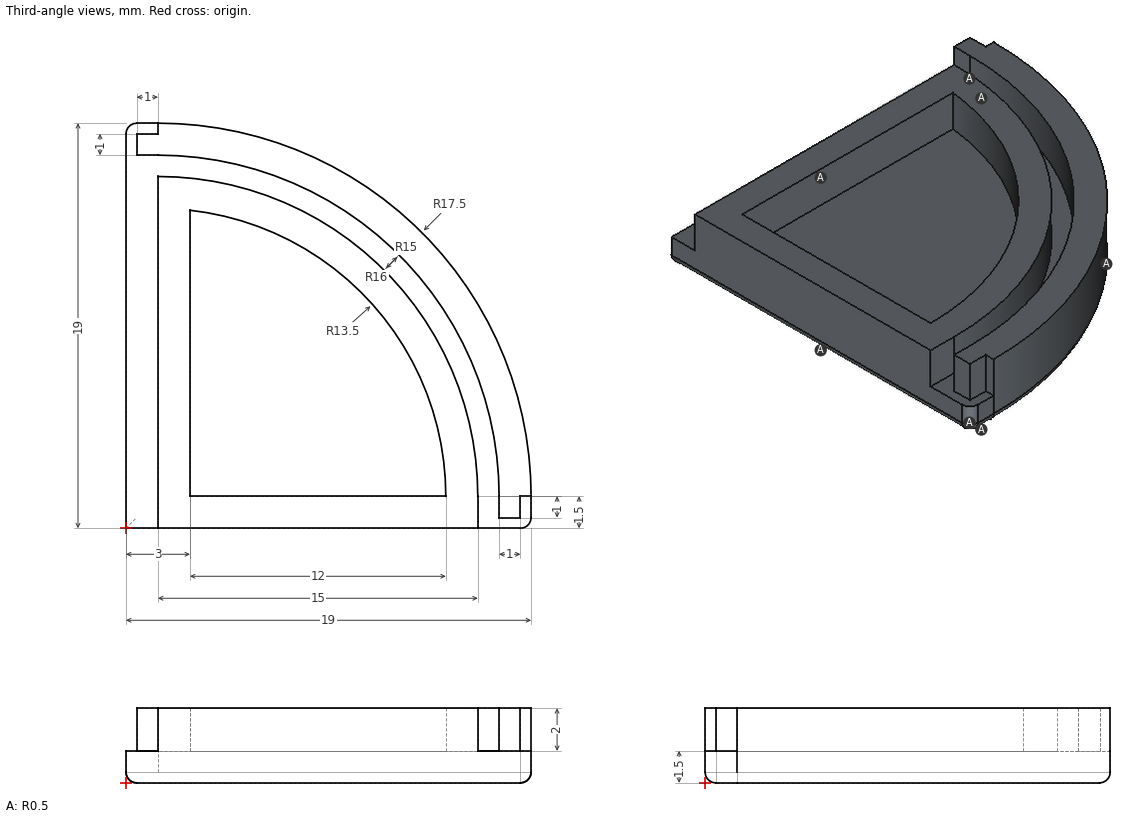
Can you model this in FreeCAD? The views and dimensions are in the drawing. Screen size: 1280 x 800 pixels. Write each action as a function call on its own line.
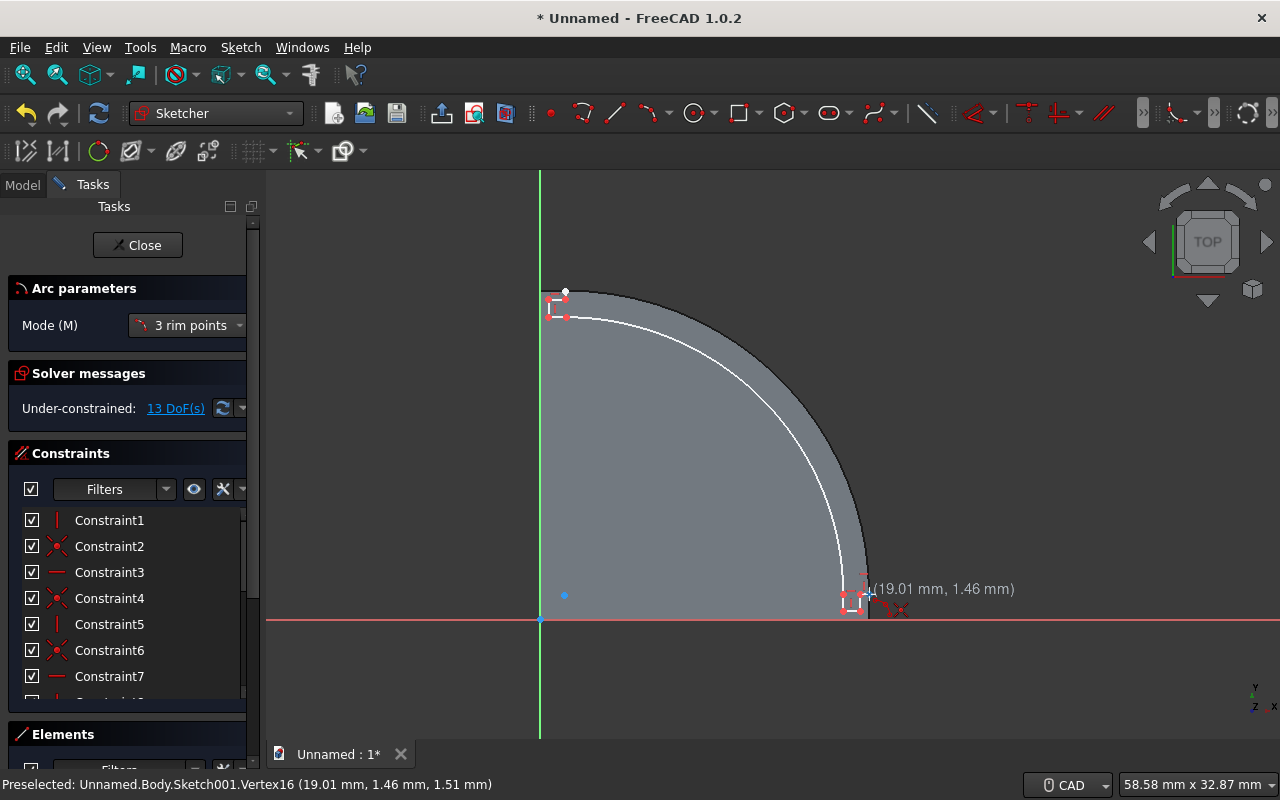
scroll(566, 291, up, 7)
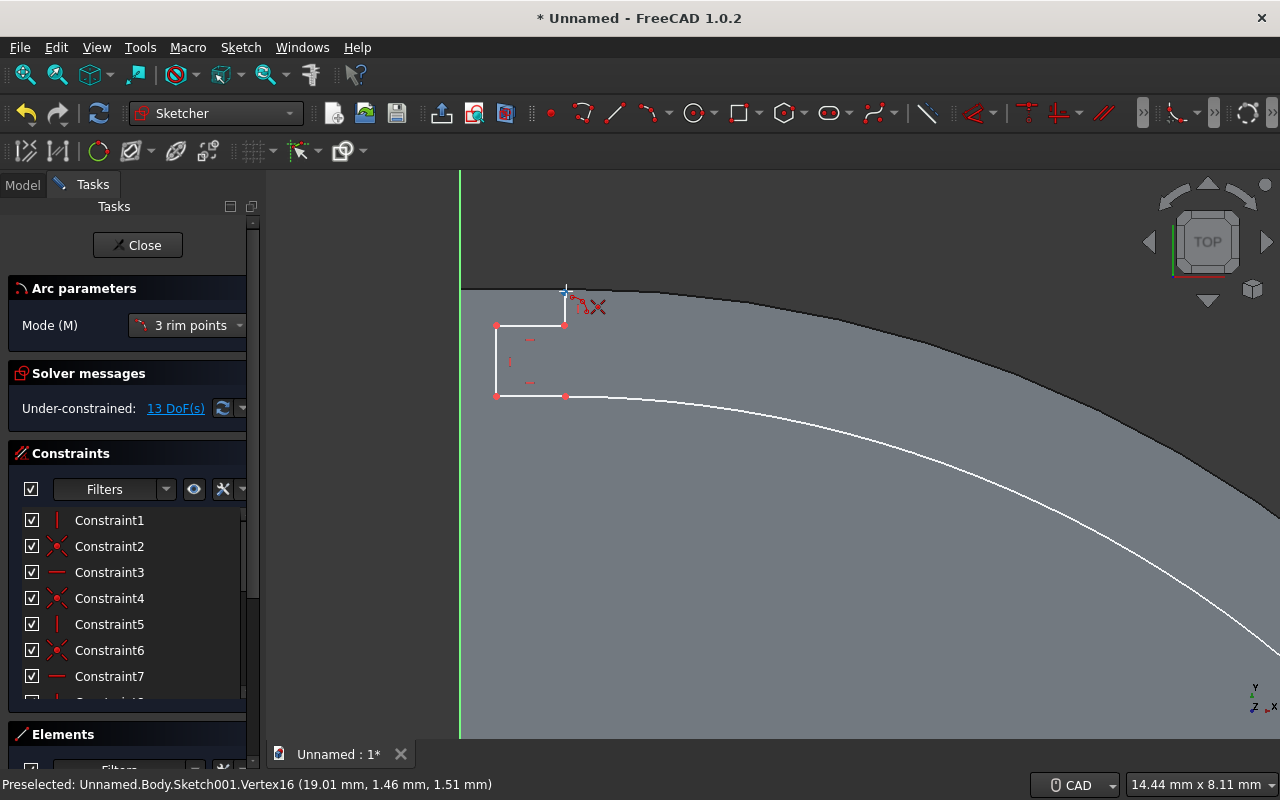
click(565, 292)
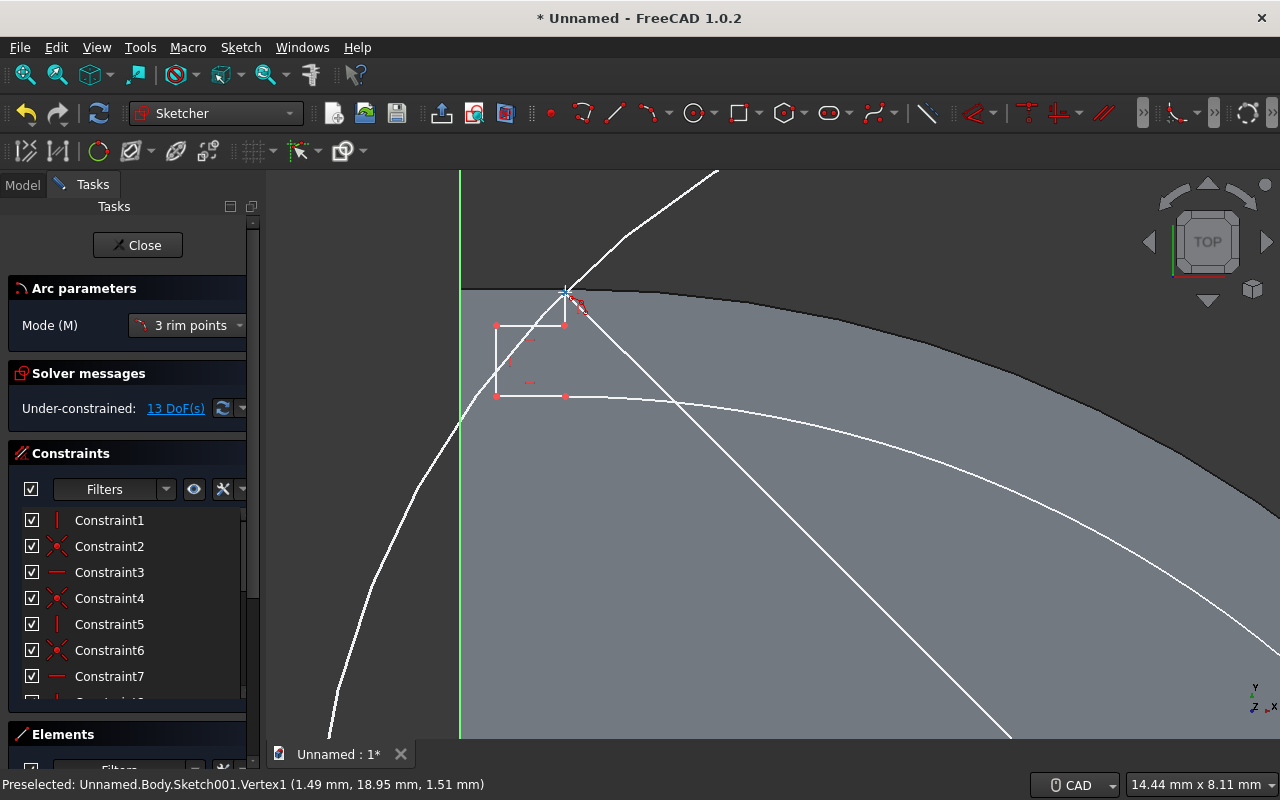
scroll(566, 290, down, 7)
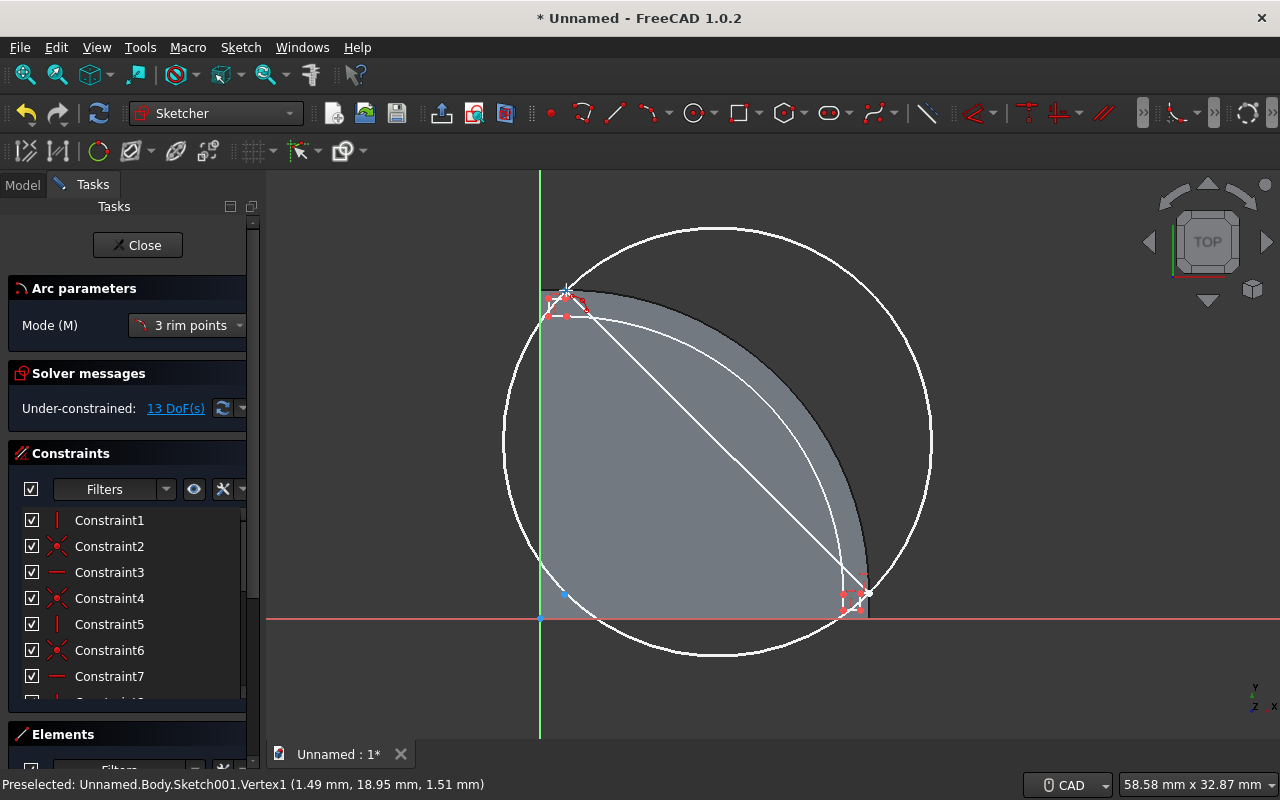
click(780, 379)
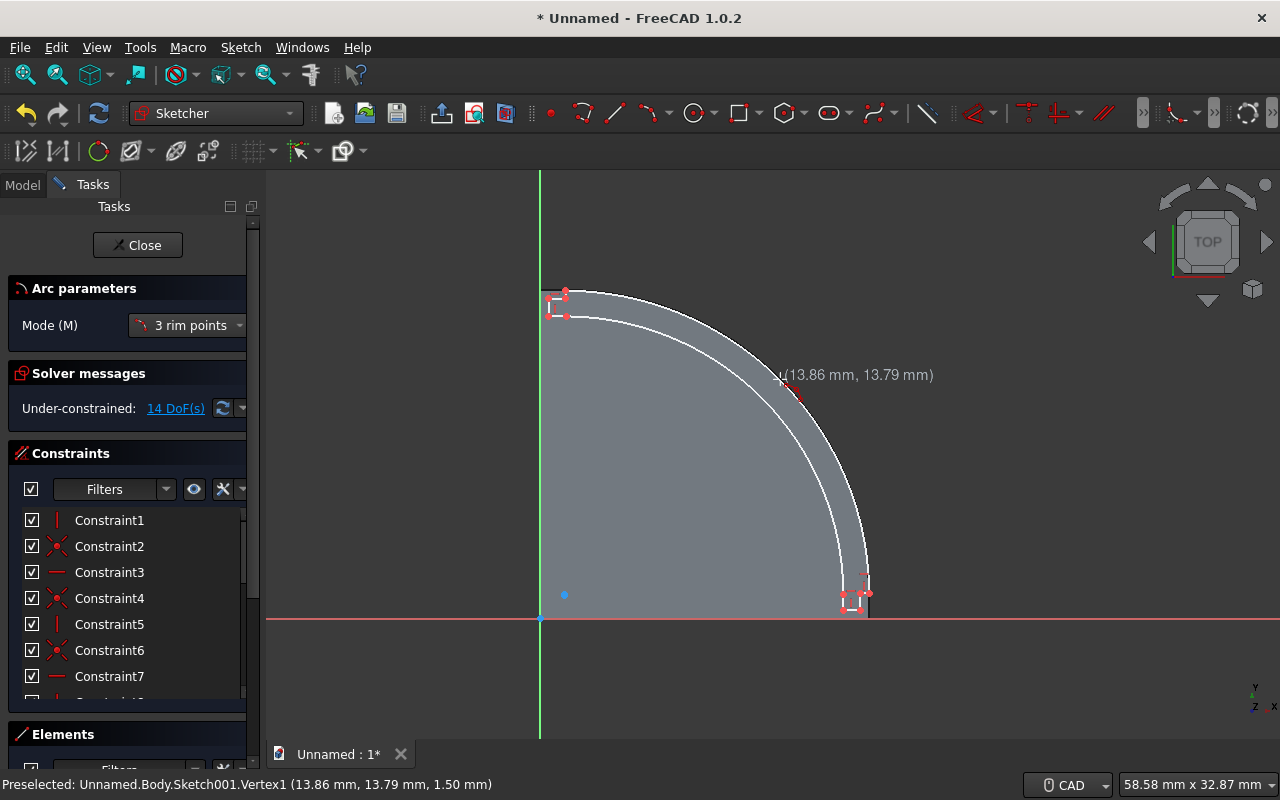
click(584, 114)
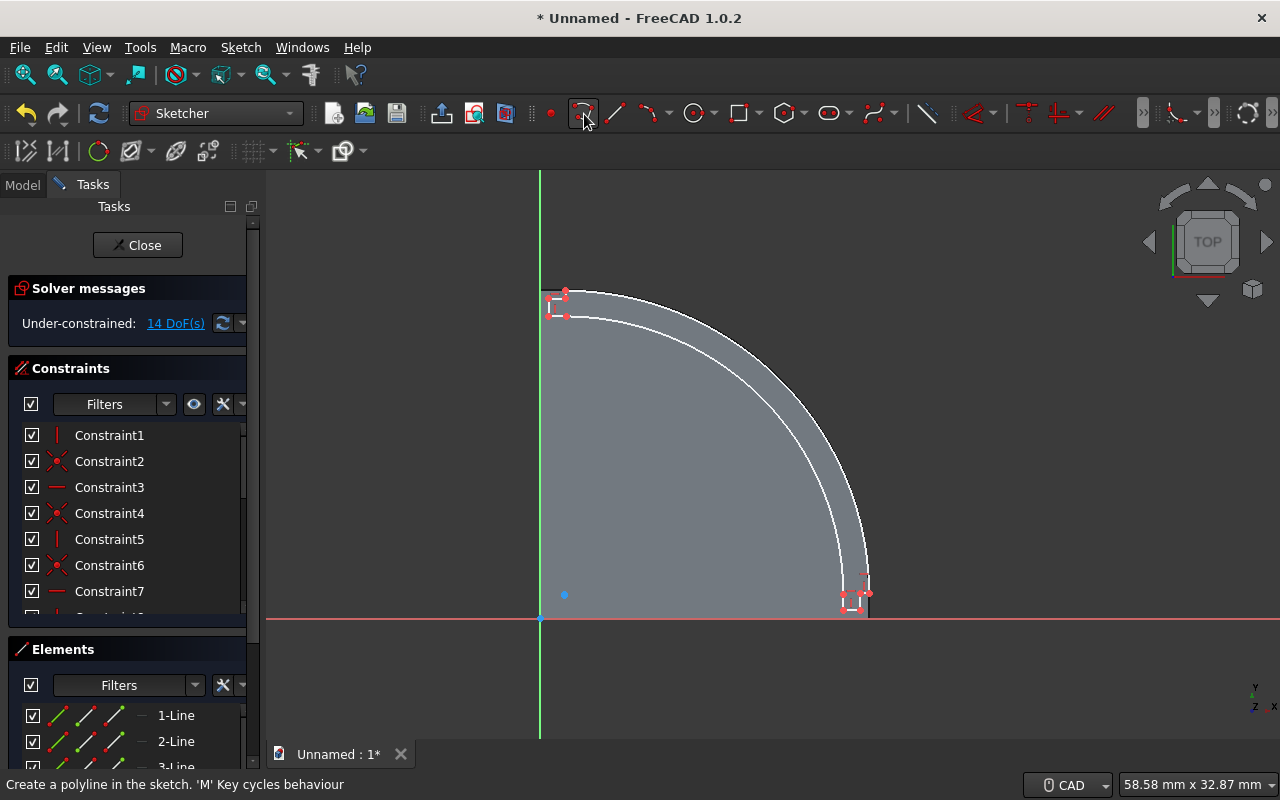
click(566, 333)
click(566, 619)
click(826, 610)
click(826, 593)
right_click(826, 593)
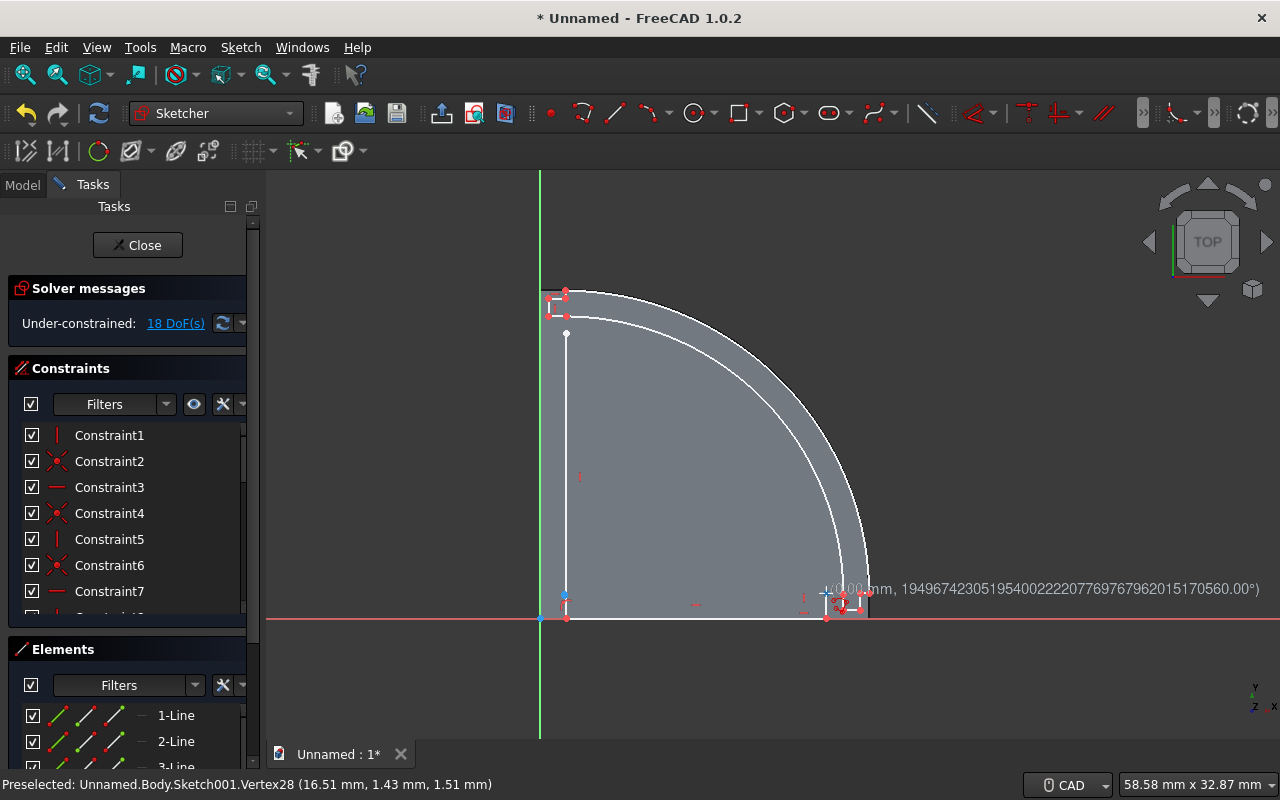
key(g)
key(3)
key(a)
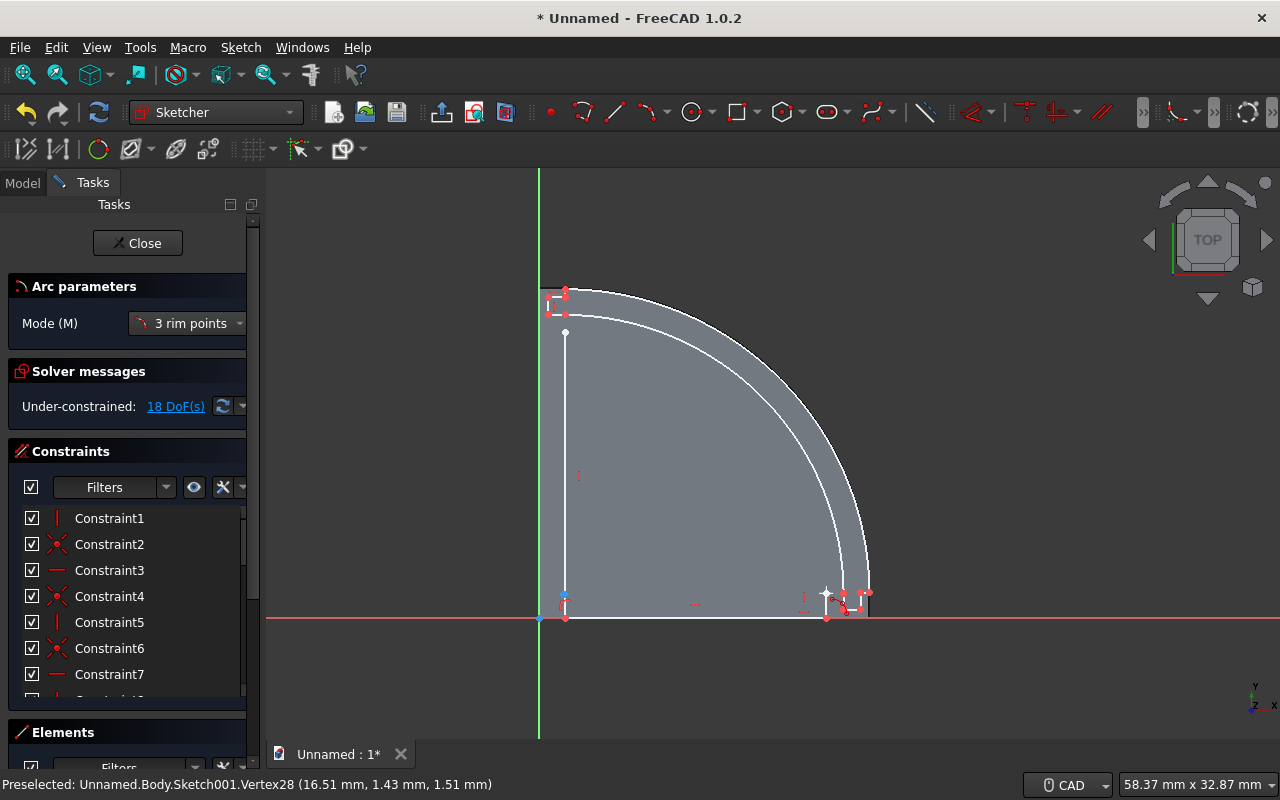
click(826, 593)
click(565, 333)
click(750, 408)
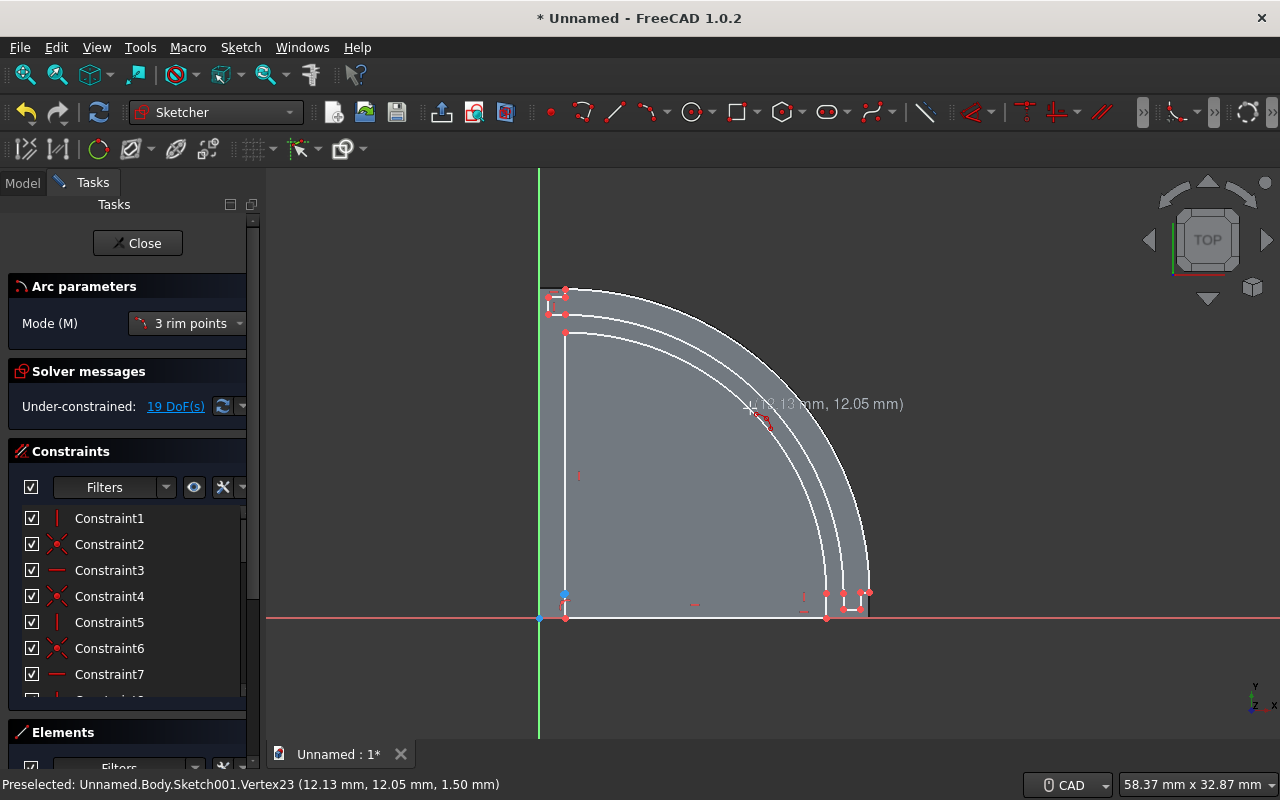
click(584, 112)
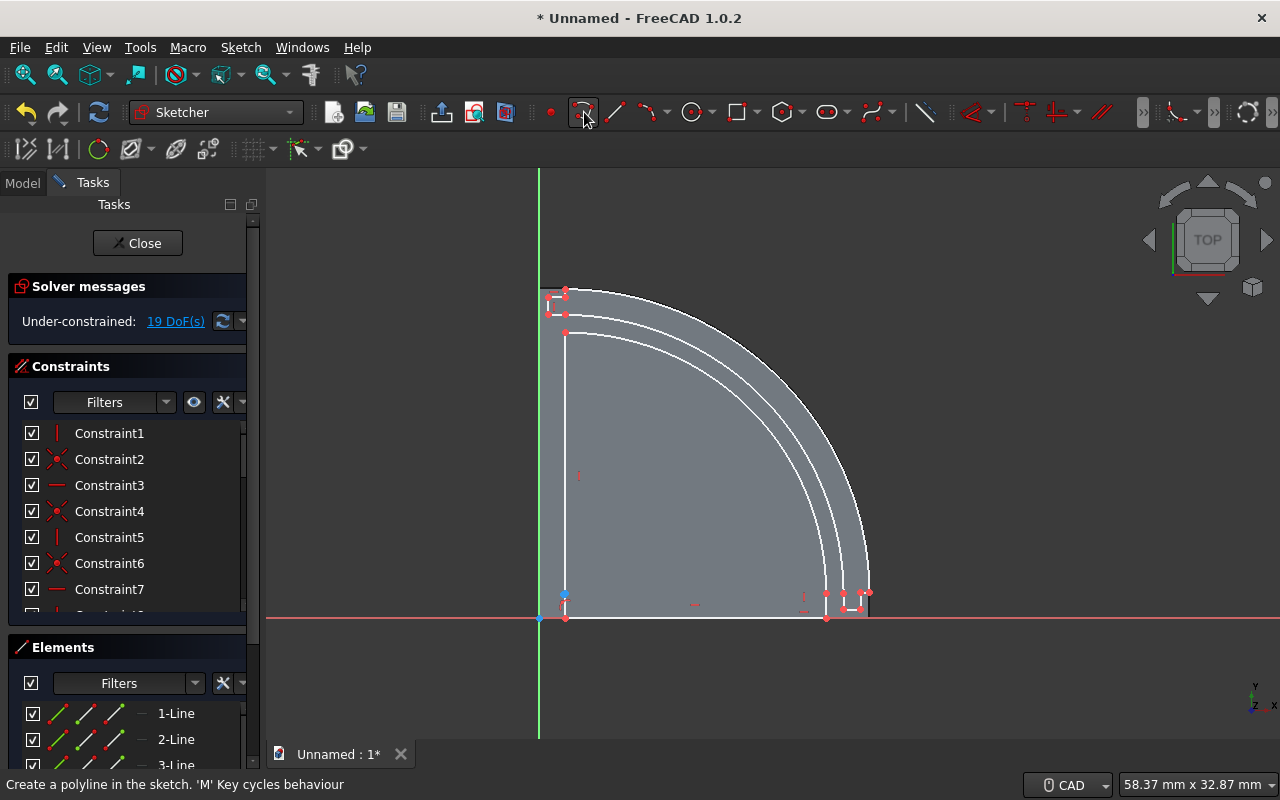
click(800, 592)
click(591, 592)
click(591, 359)
right_click(591, 359)